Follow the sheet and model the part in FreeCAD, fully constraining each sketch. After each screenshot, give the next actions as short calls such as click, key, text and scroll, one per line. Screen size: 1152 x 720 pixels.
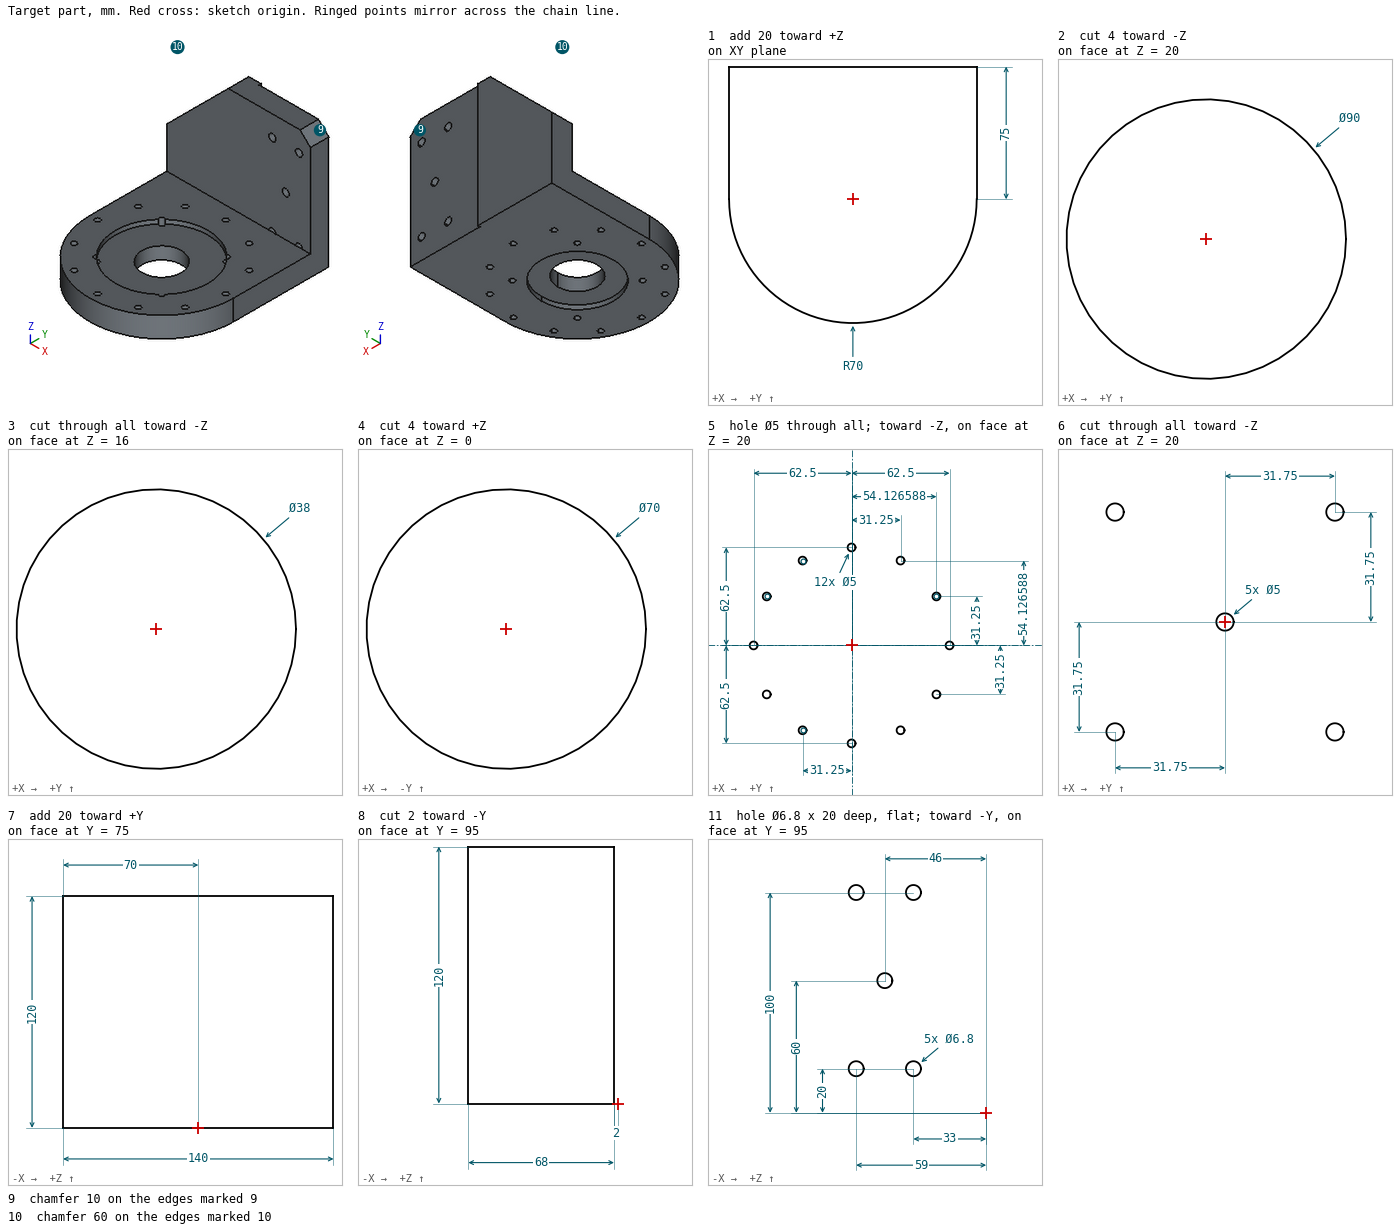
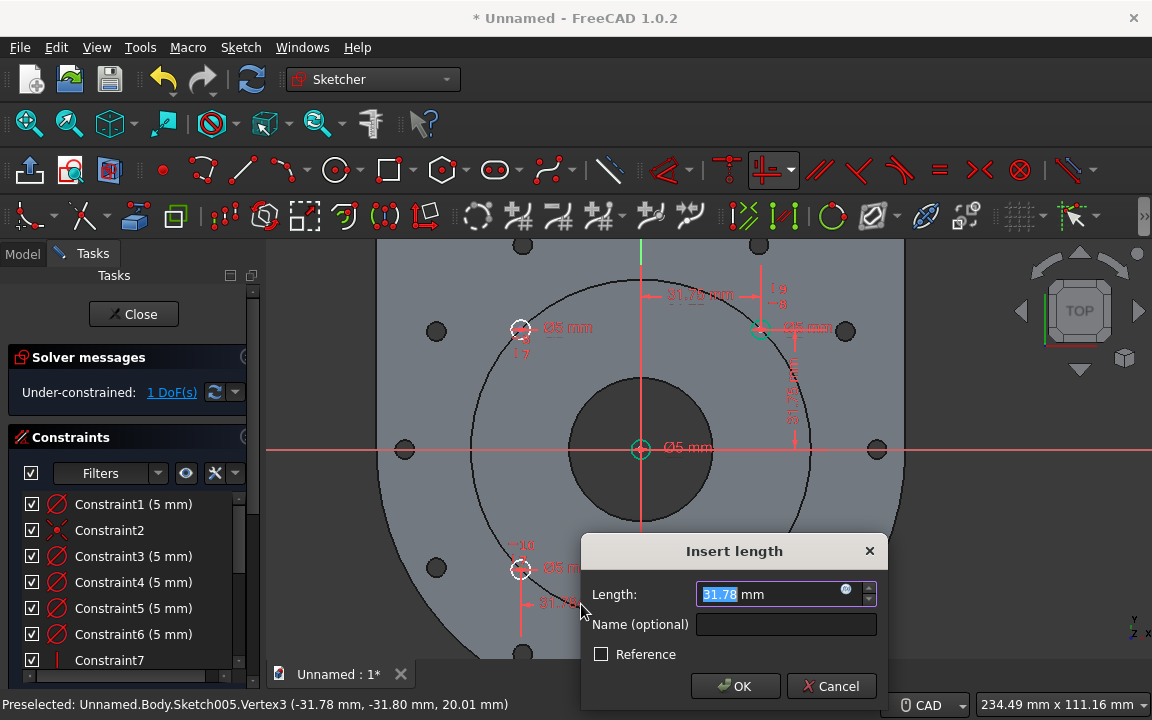
text(31.75)
key(Return)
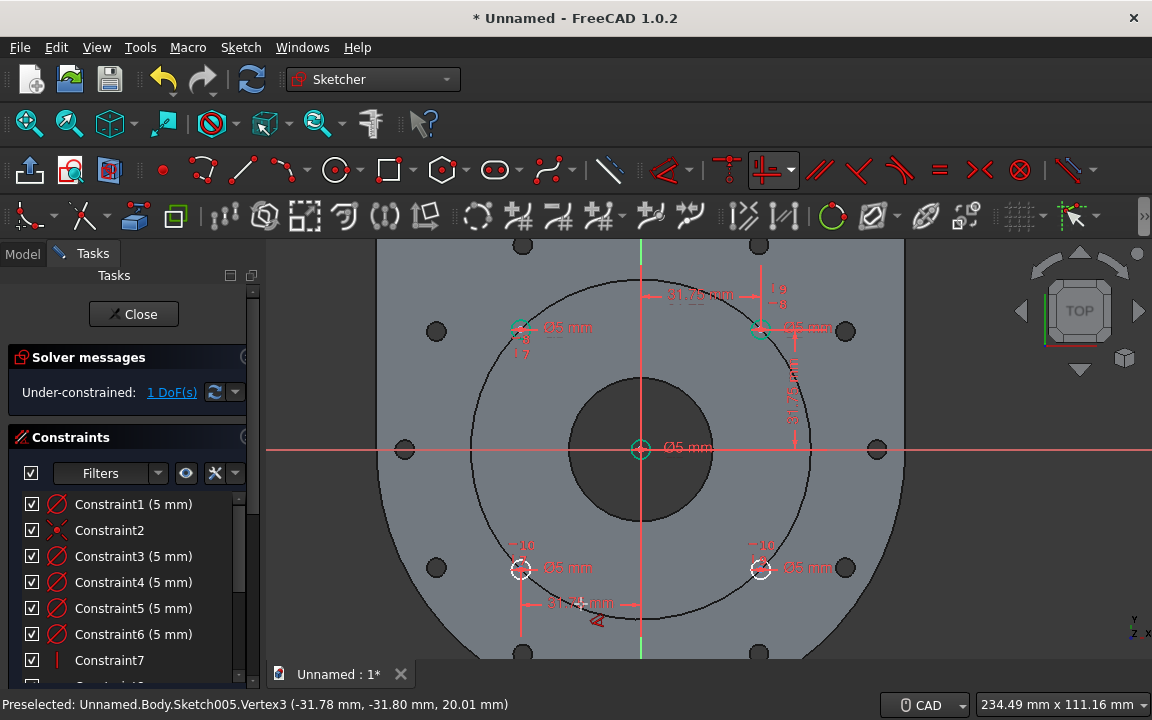
click(521, 570)
click(487, 510)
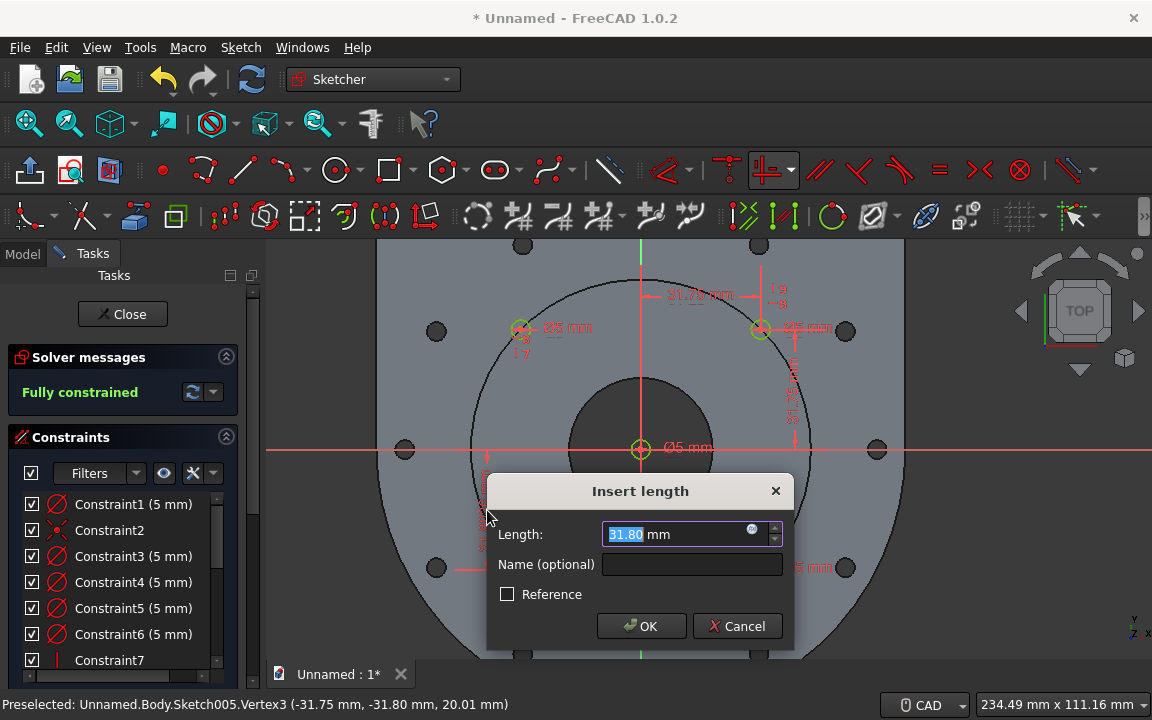
text(31.75)
key(Return)
key(Escape)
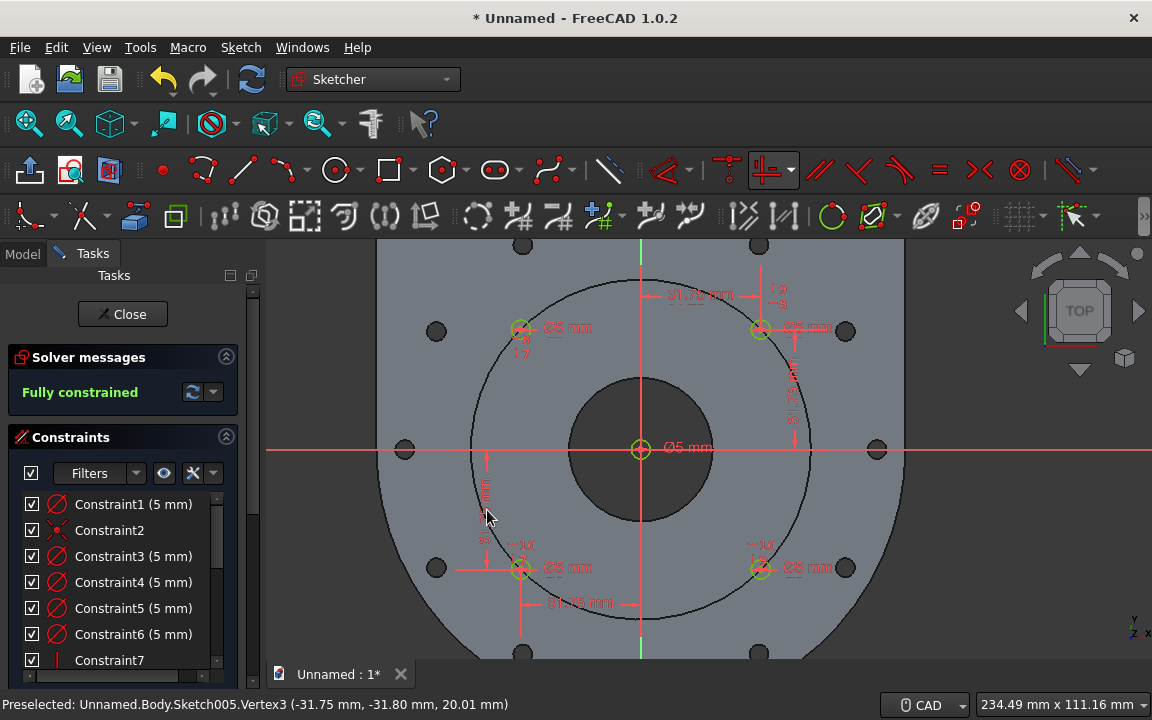
click(123, 314)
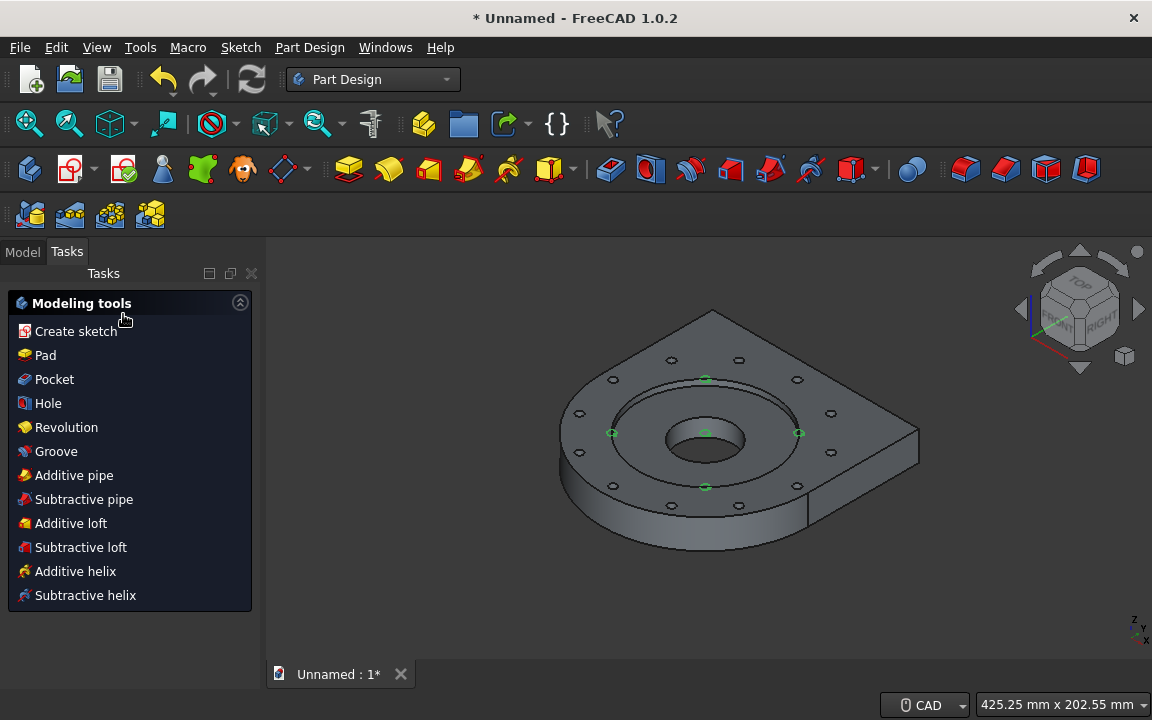
click(612, 170)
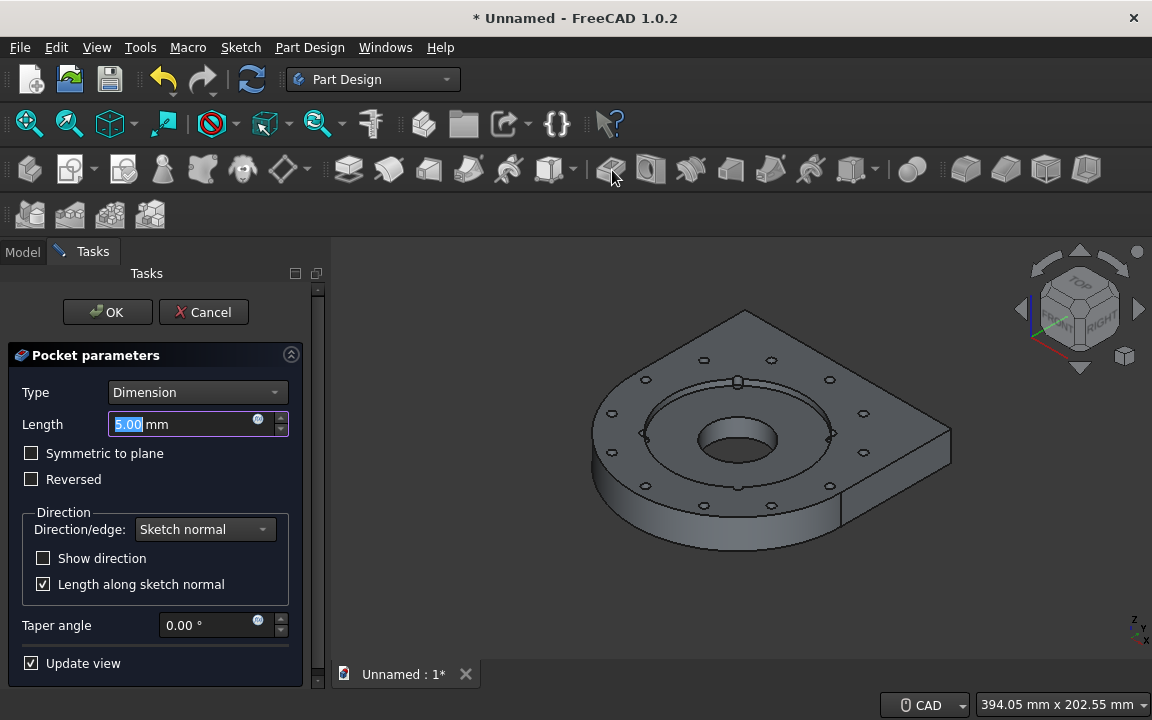
click(198, 392)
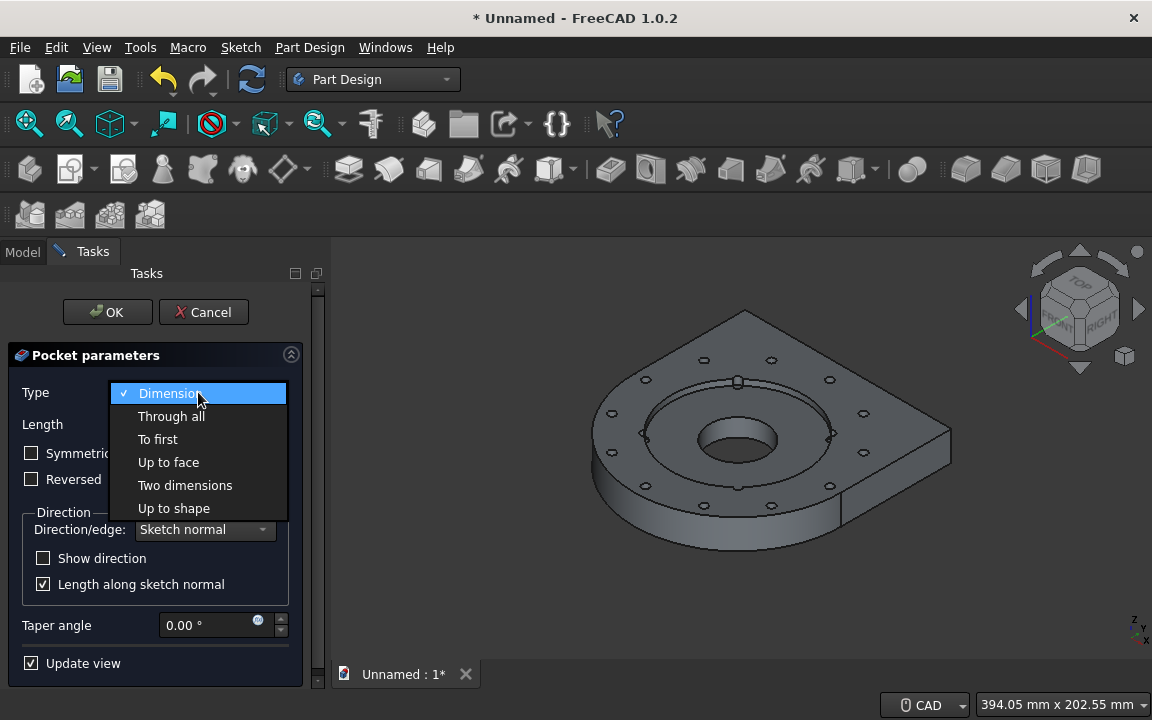
click(198, 416)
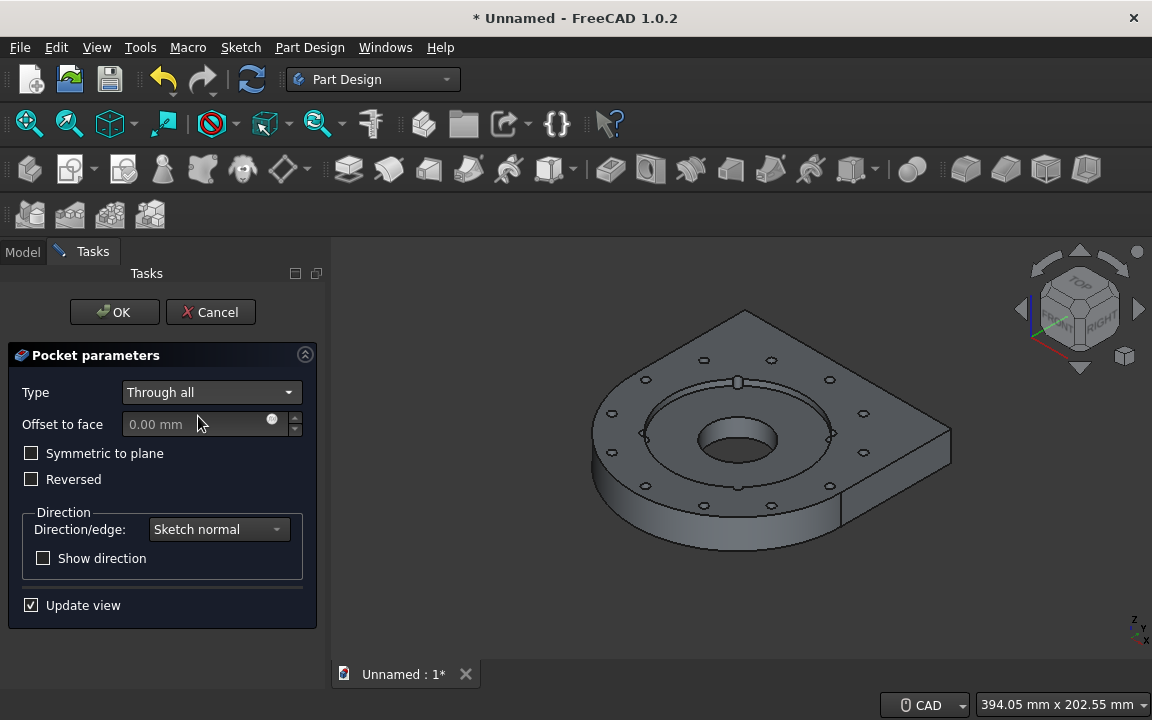
click(115, 312)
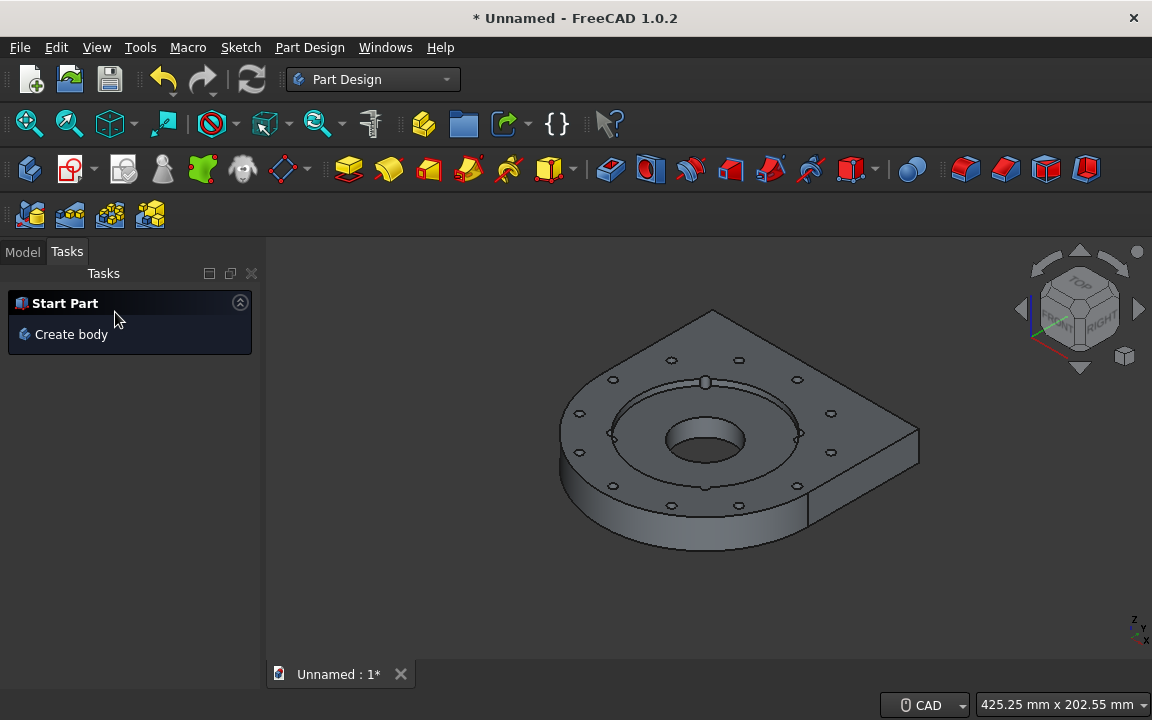
key(4)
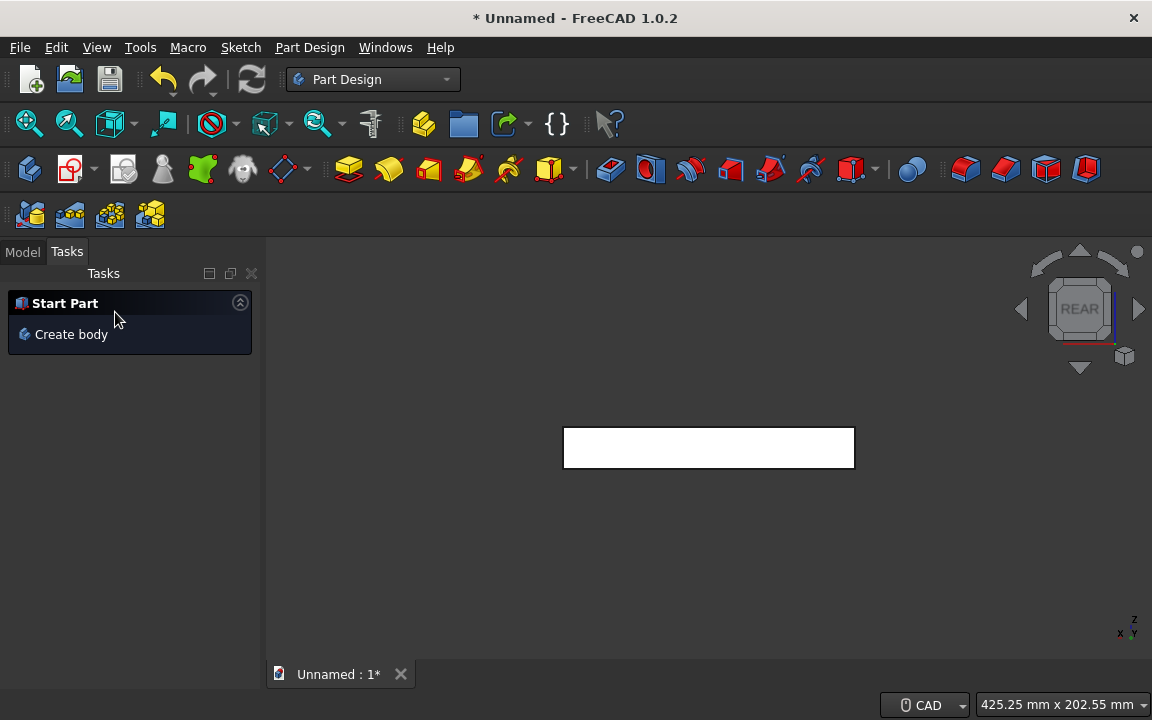
click(30, 124)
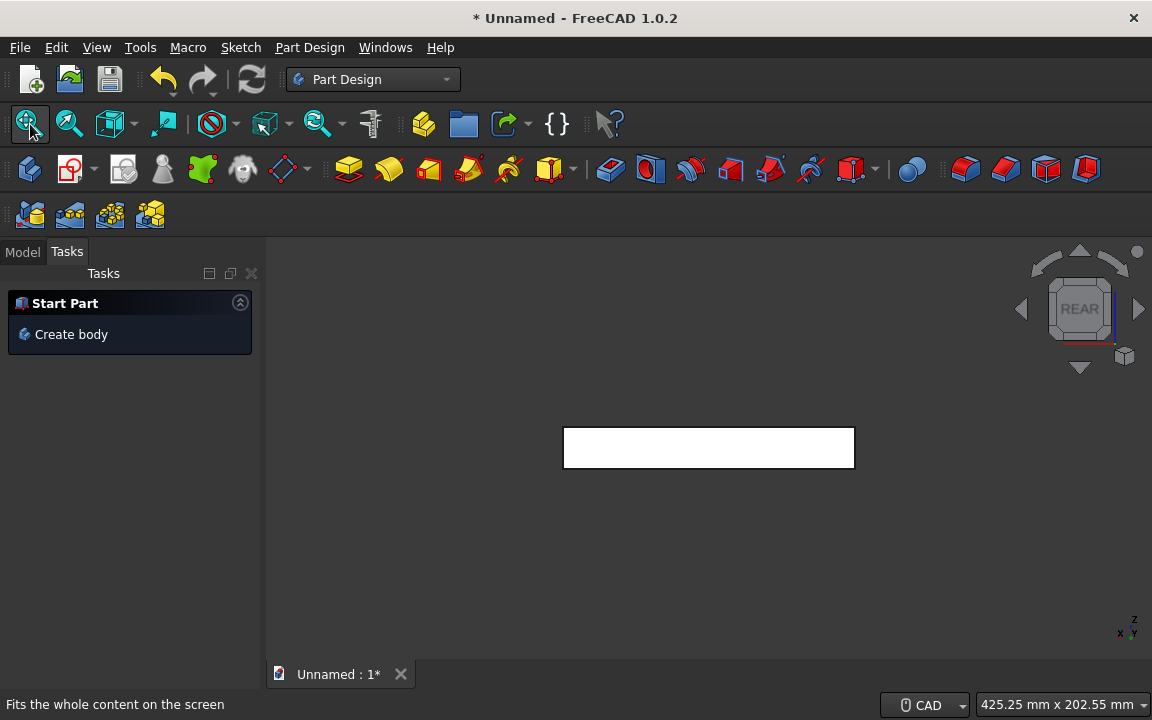
click(584, 447)